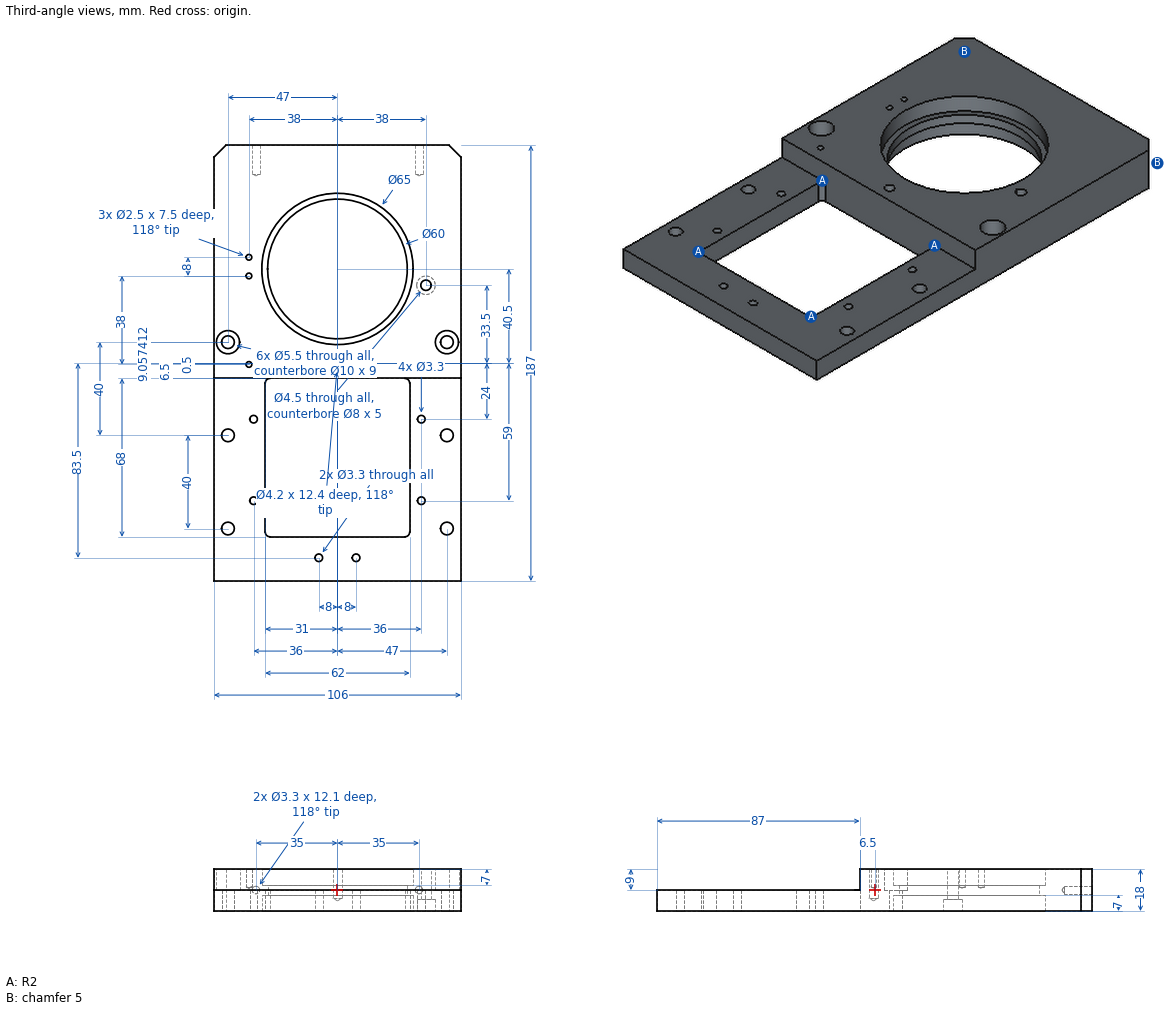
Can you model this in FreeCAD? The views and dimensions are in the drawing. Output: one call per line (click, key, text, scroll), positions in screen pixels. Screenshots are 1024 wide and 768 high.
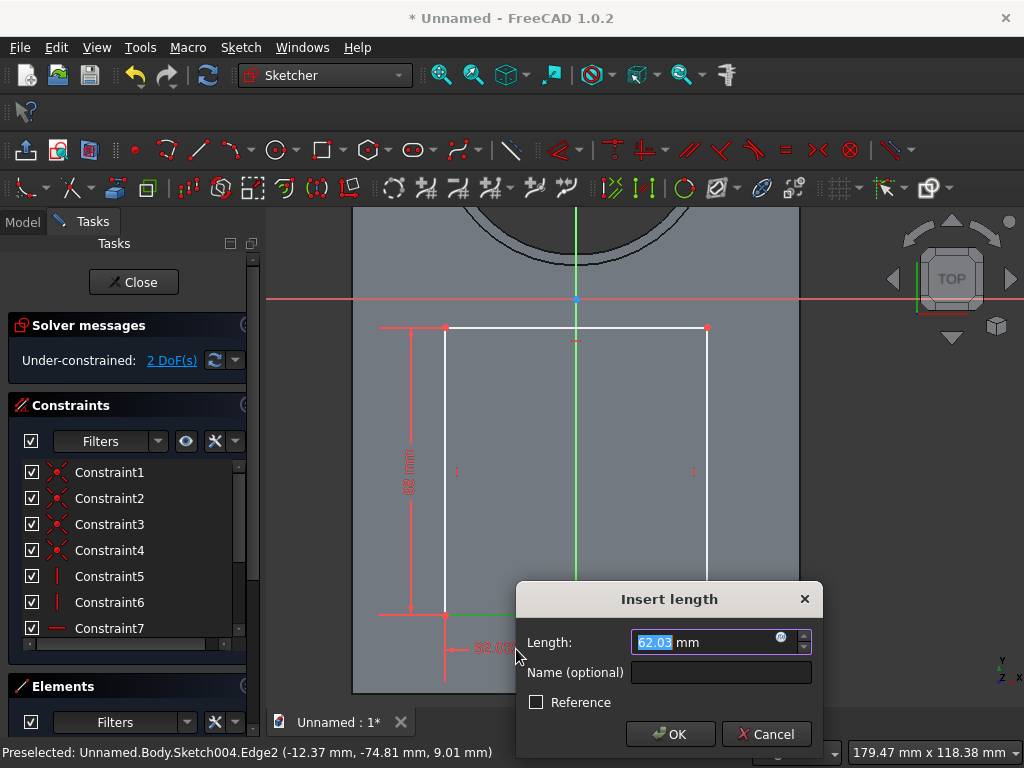
text(62)
key(Return)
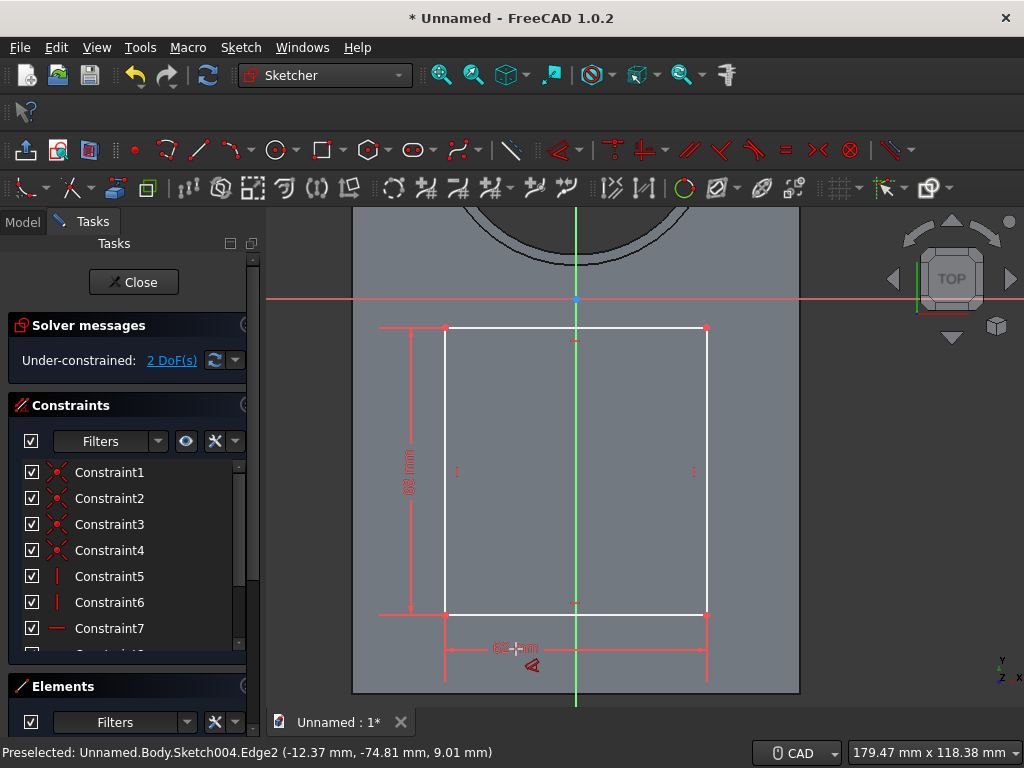
click(445, 328)
click(511, 265)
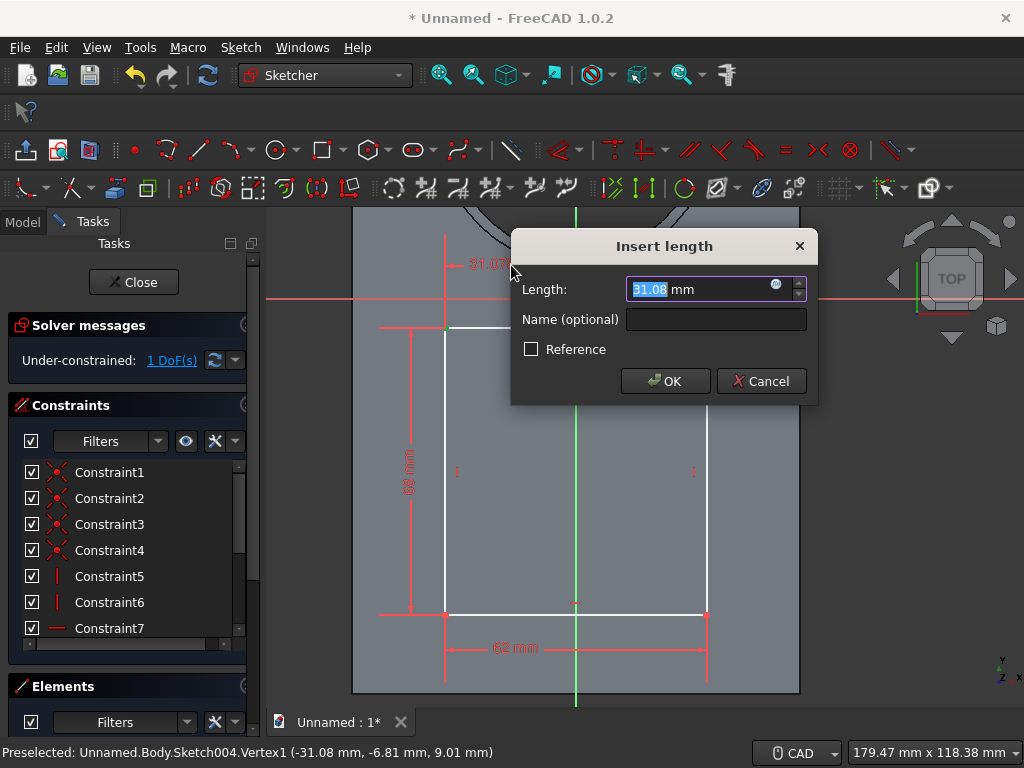
text(31)
key(Return)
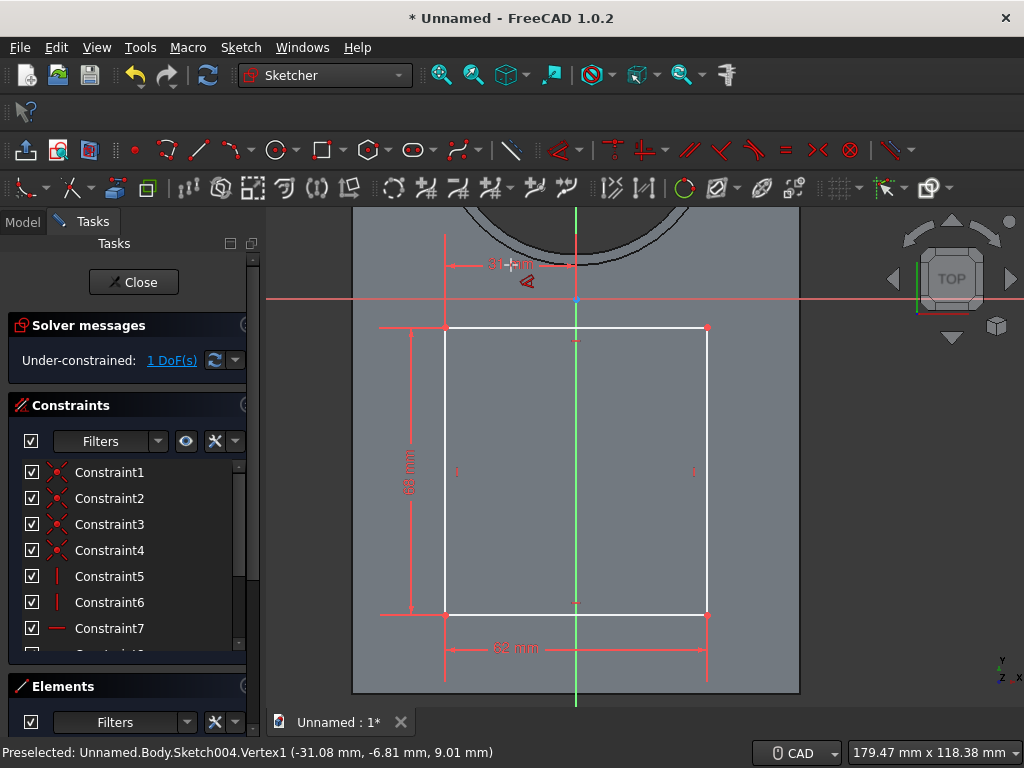
scroll(445, 328, up, 2)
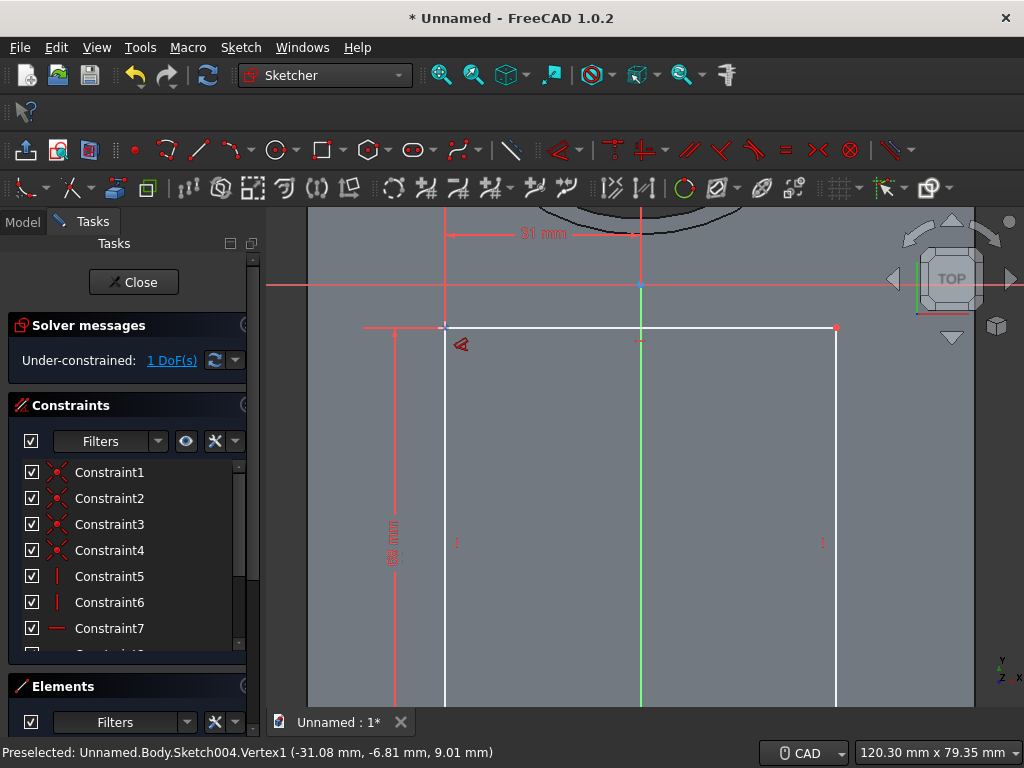
click(445, 328)
click(411, 306)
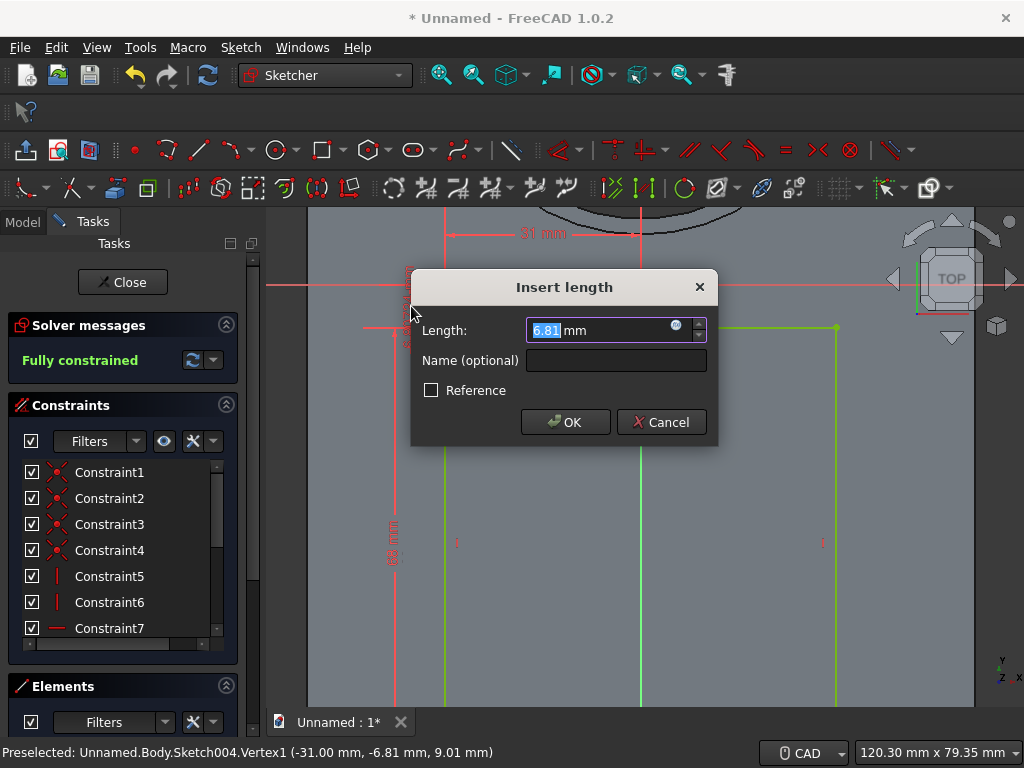
text(6.5)
key(Return)
key(Escape)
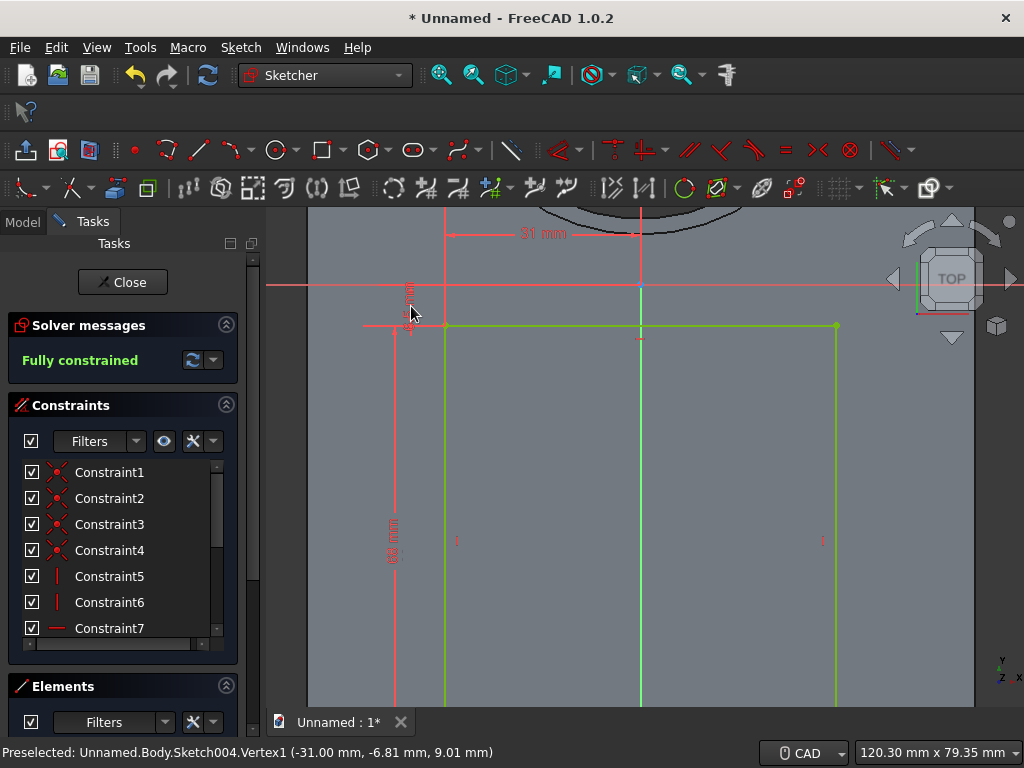
click(123, 282)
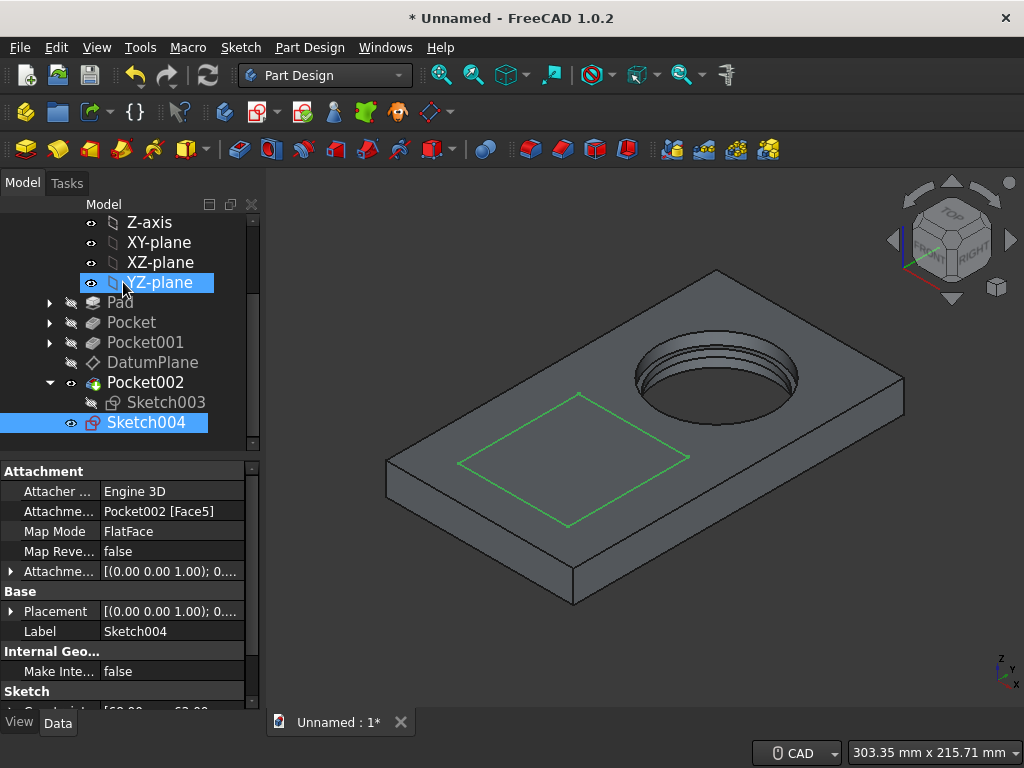
click(240, 150)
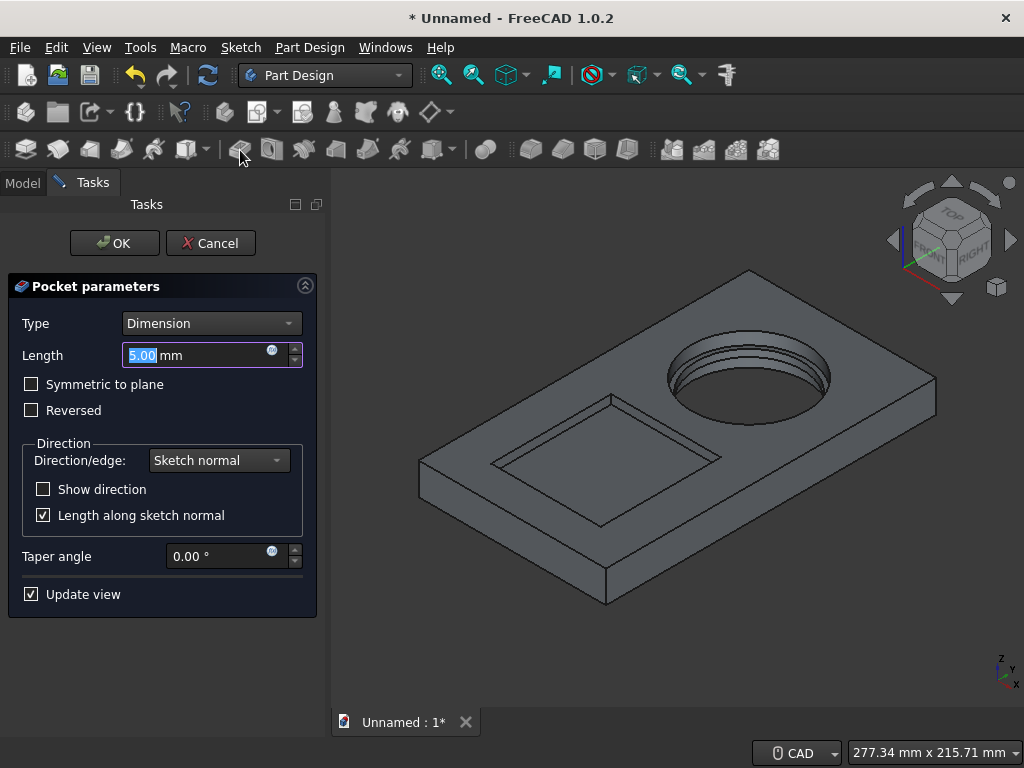
click(212, 324)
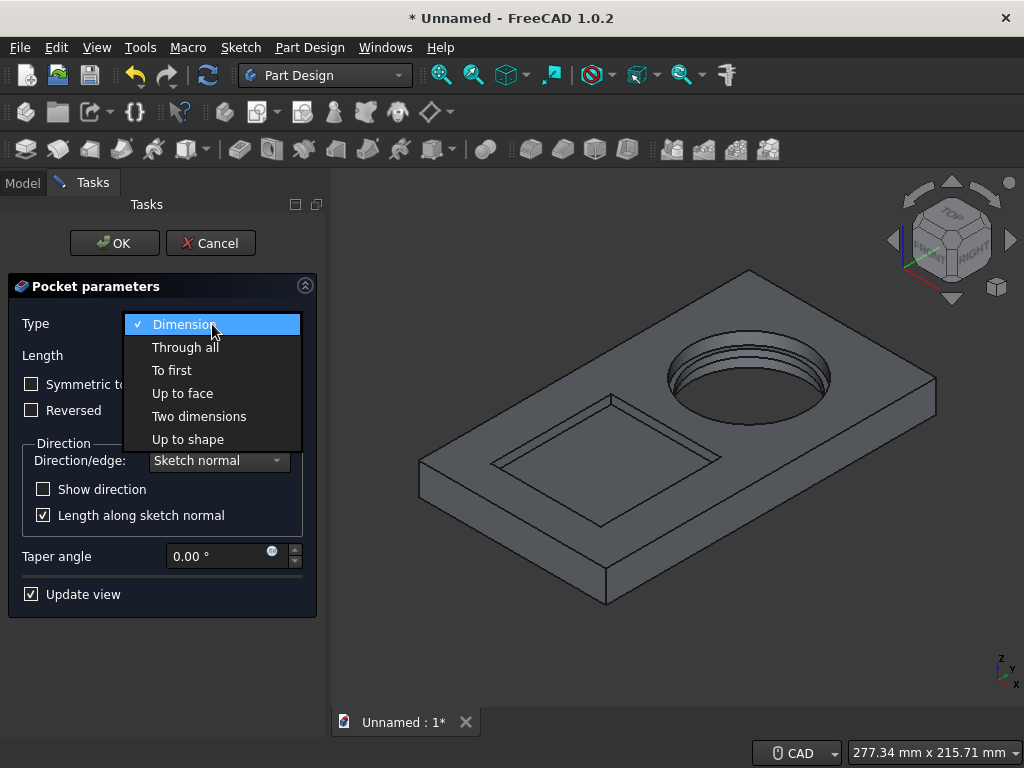
click(212, 348)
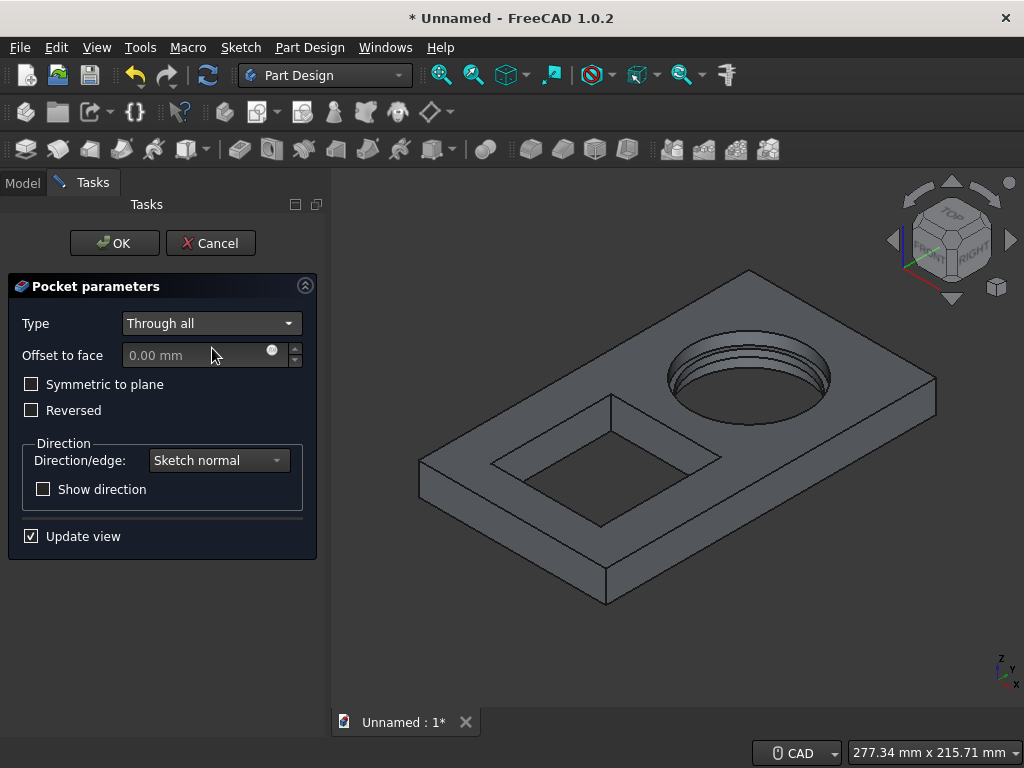
click(115, 243)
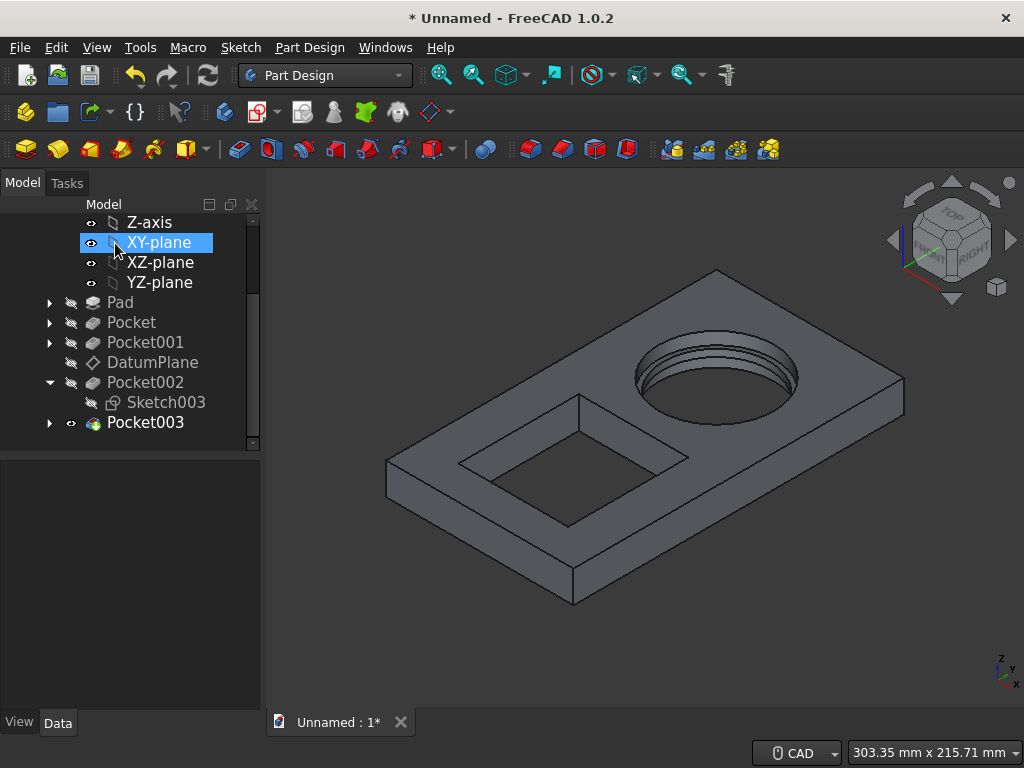
key(2)